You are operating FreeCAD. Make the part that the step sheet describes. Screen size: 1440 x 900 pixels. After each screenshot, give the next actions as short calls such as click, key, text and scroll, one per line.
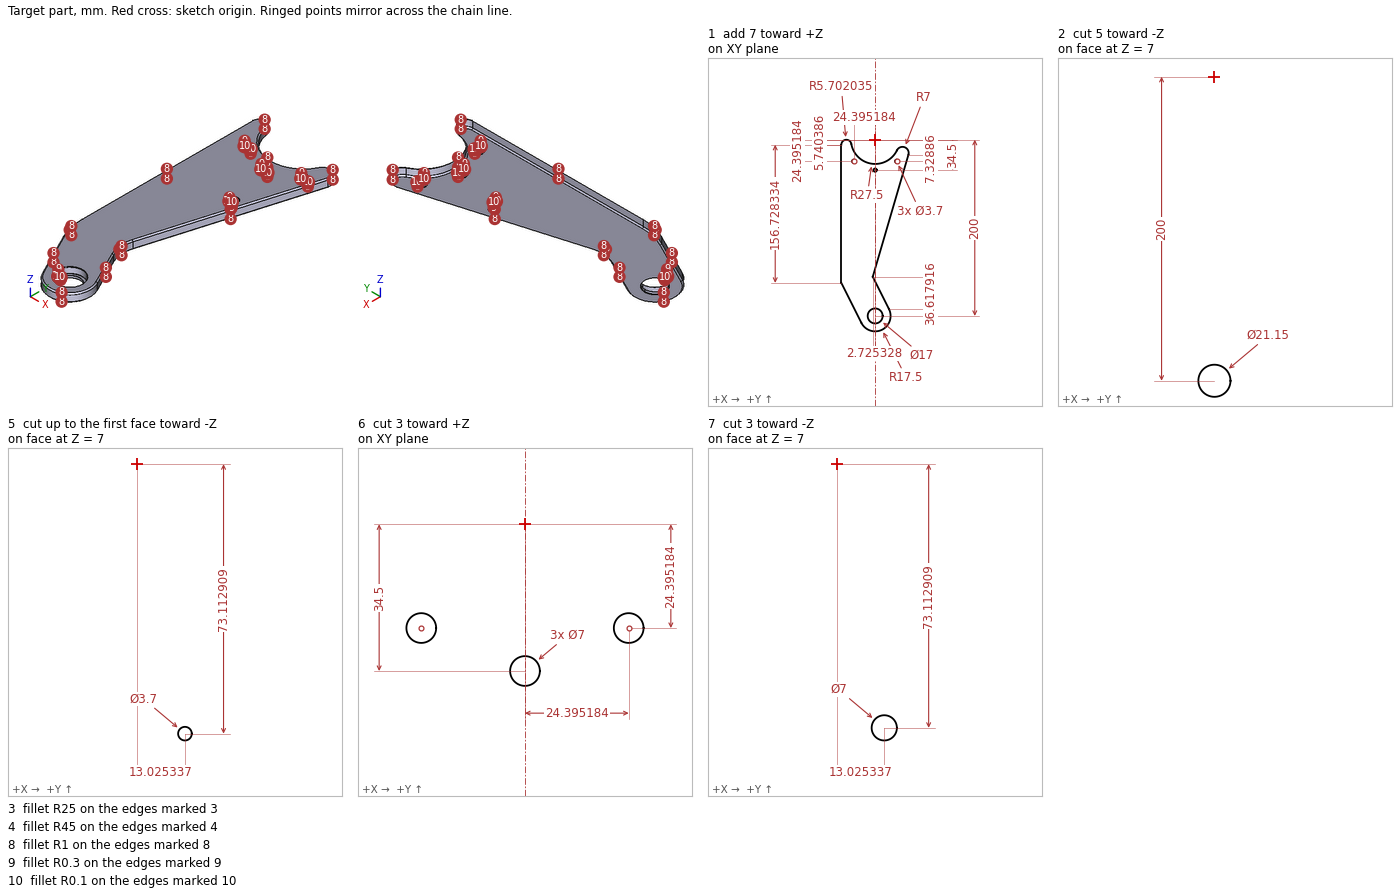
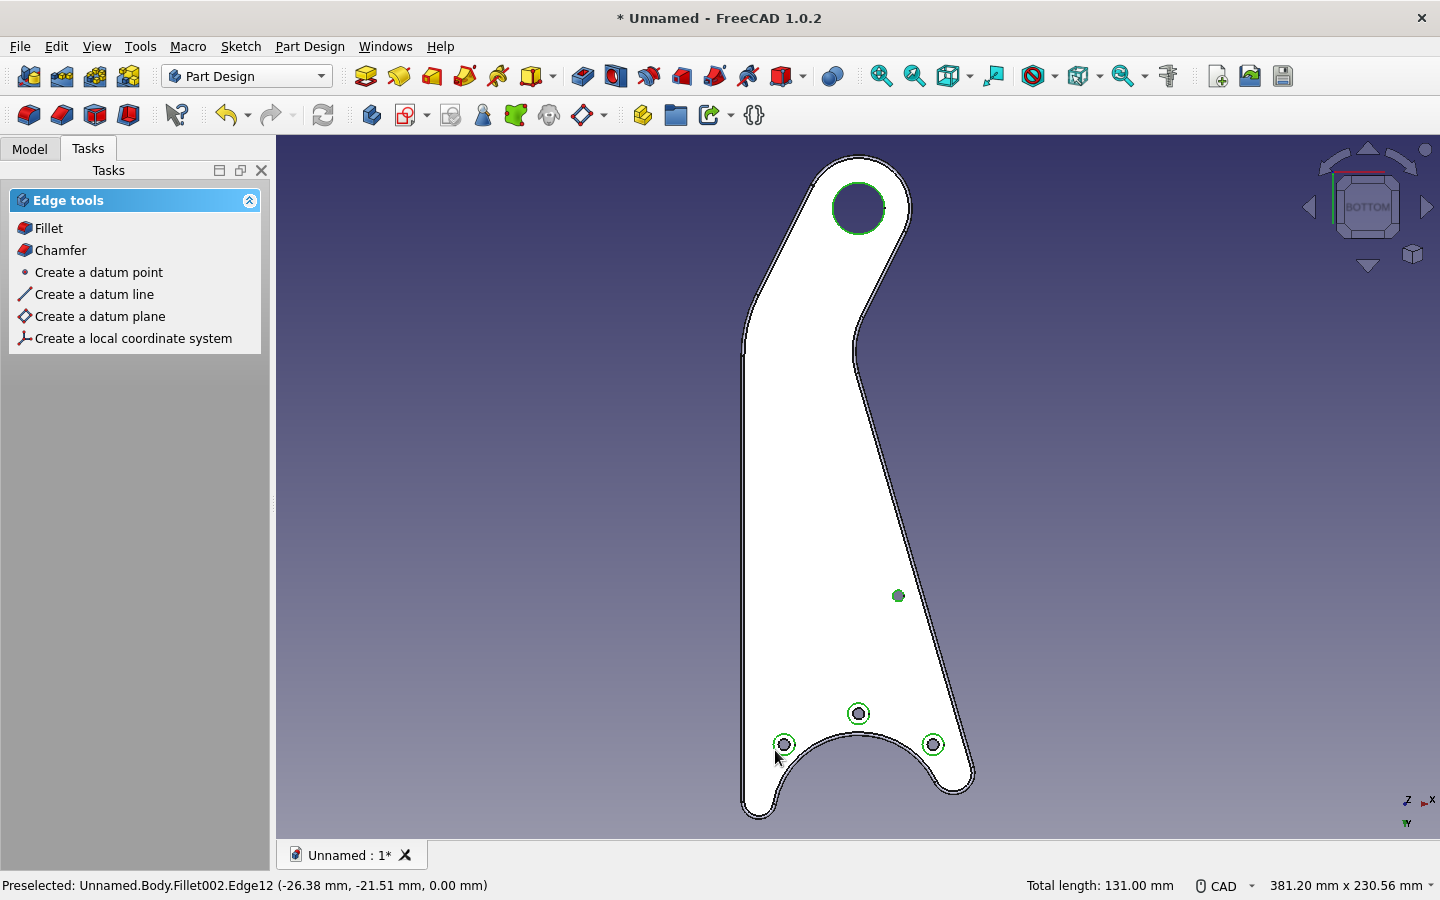
key(0)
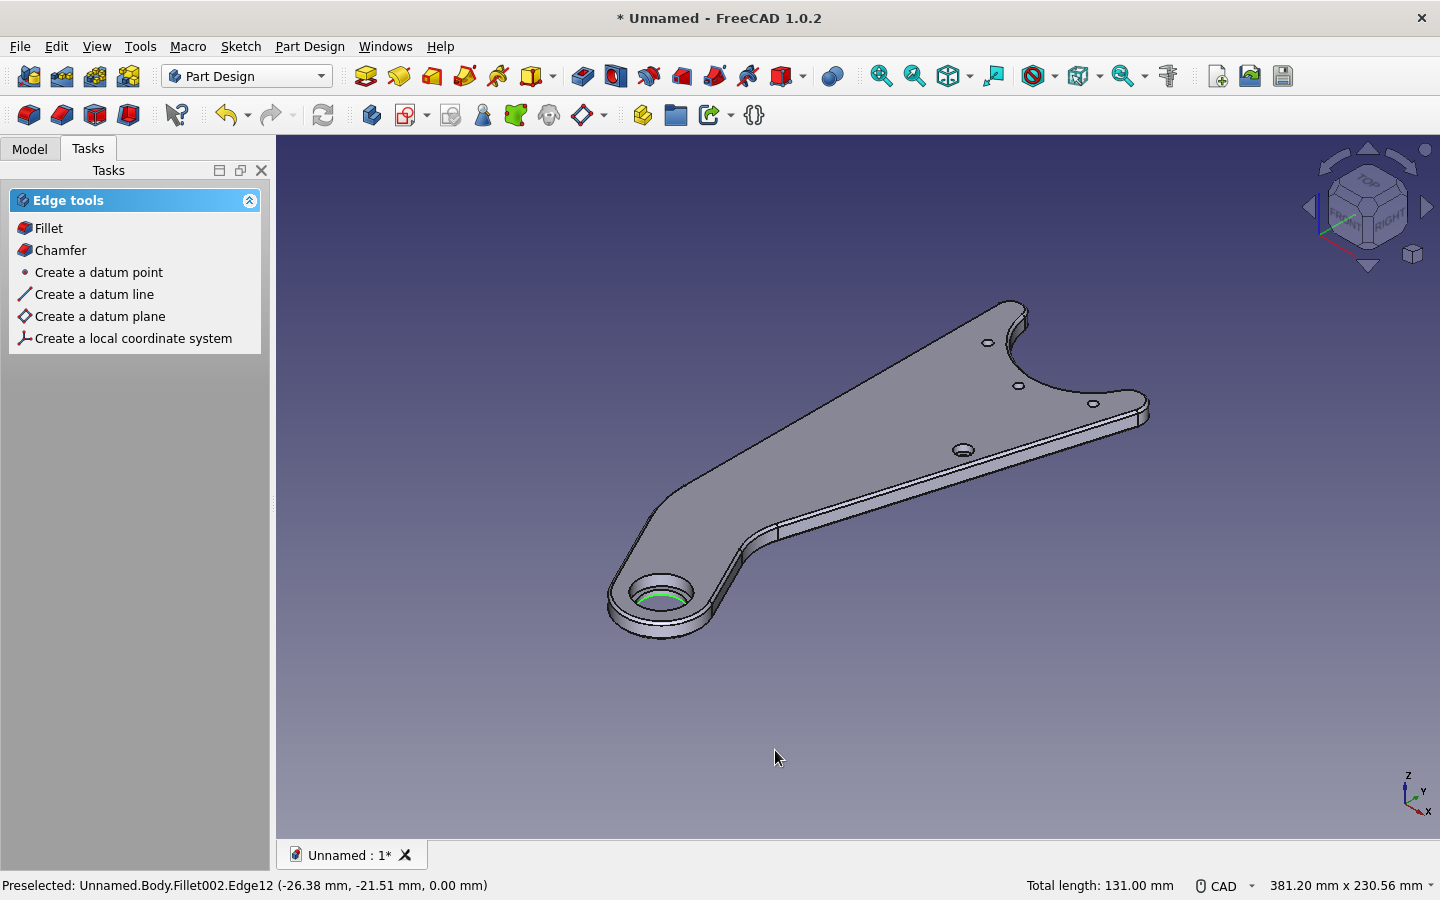
click(984, 340, ctrl)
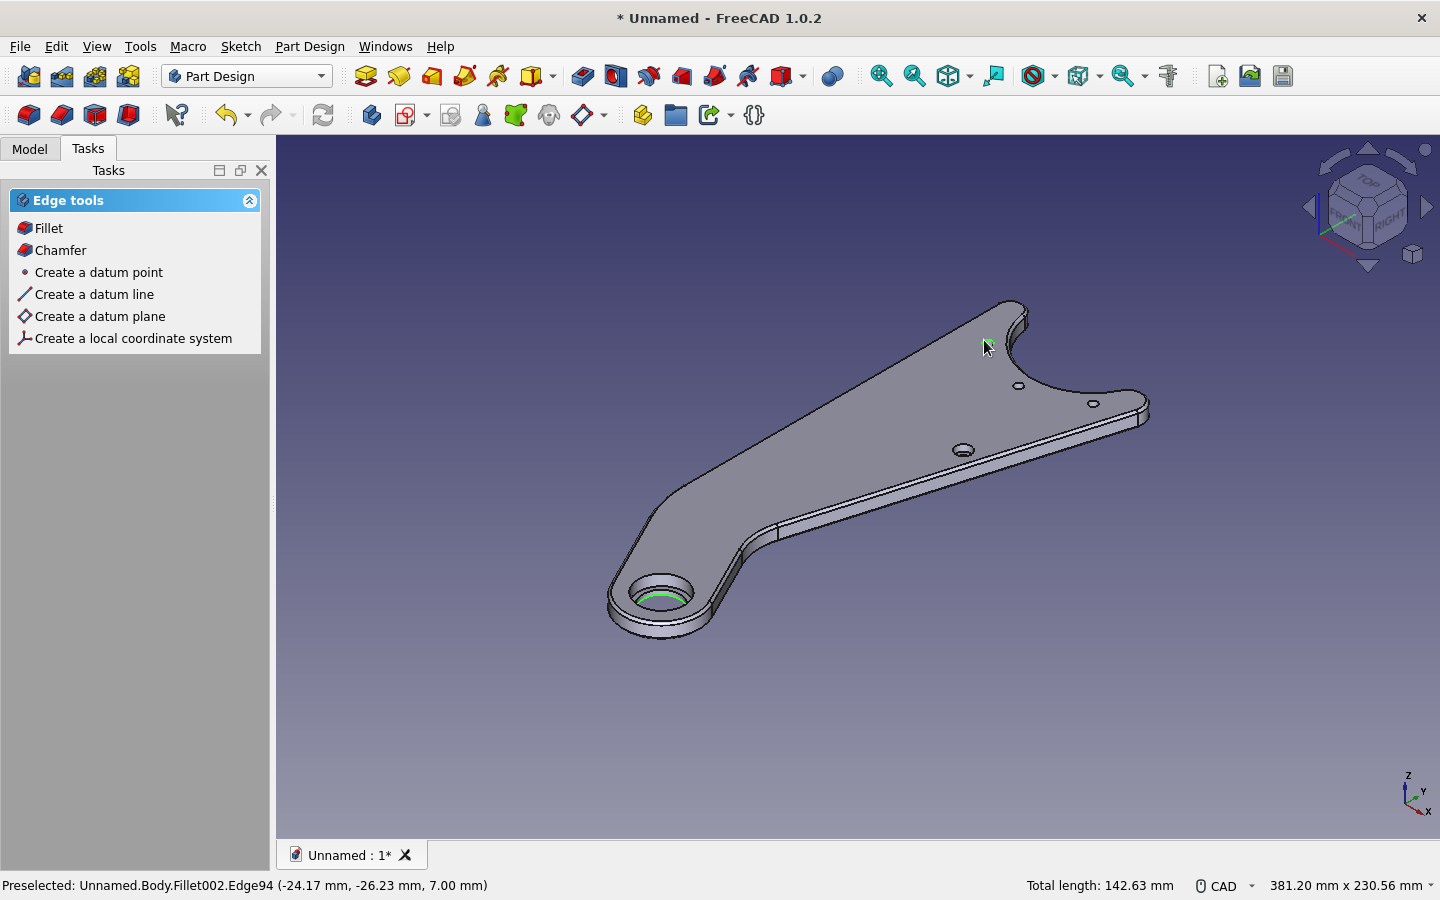
click(1089, 400, ctrl)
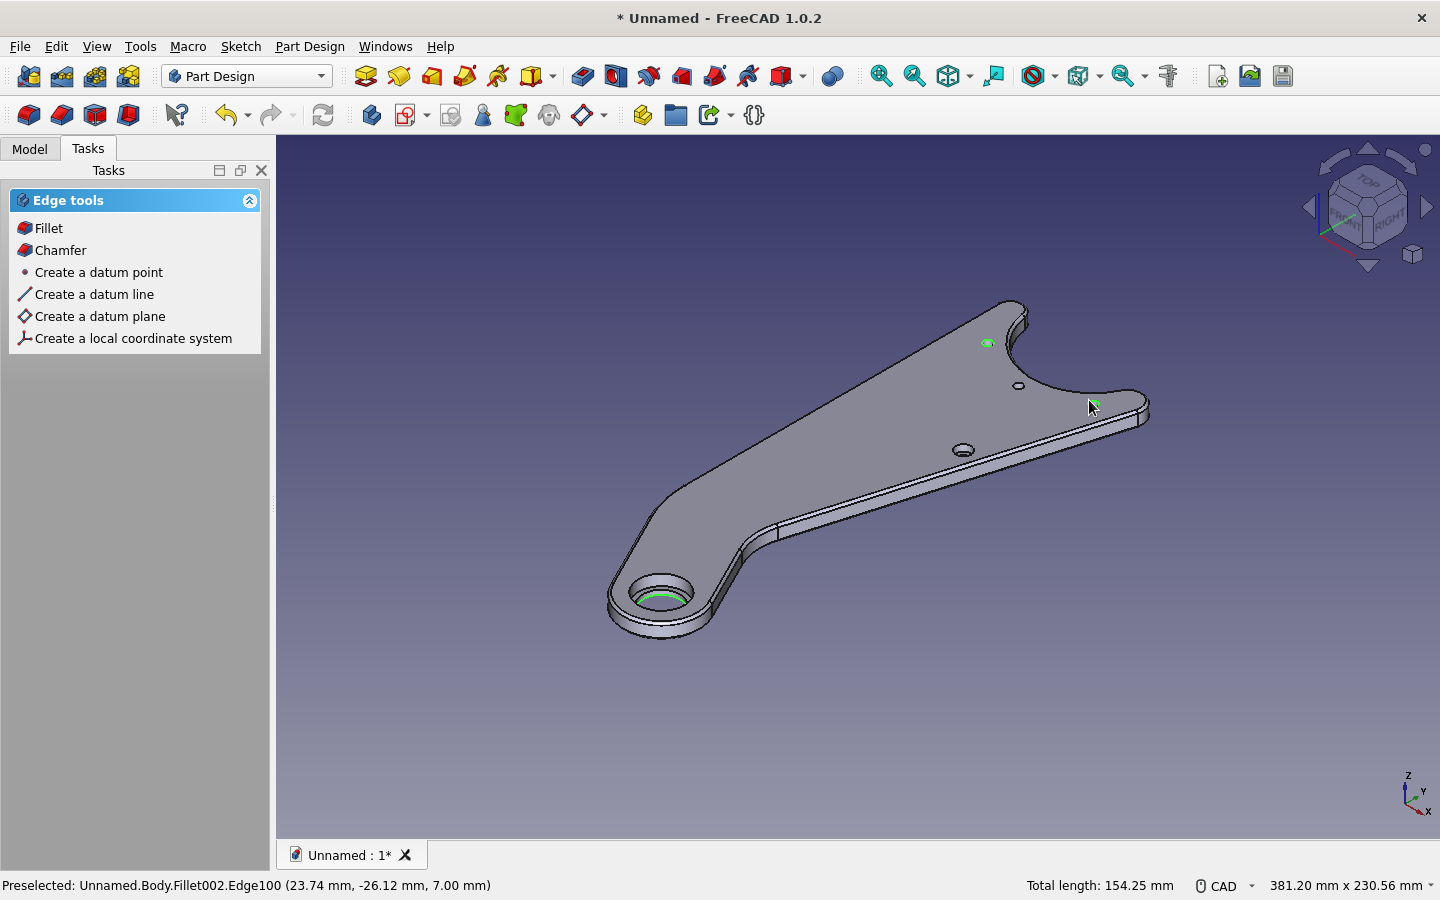
click(1015, 383, ctrl)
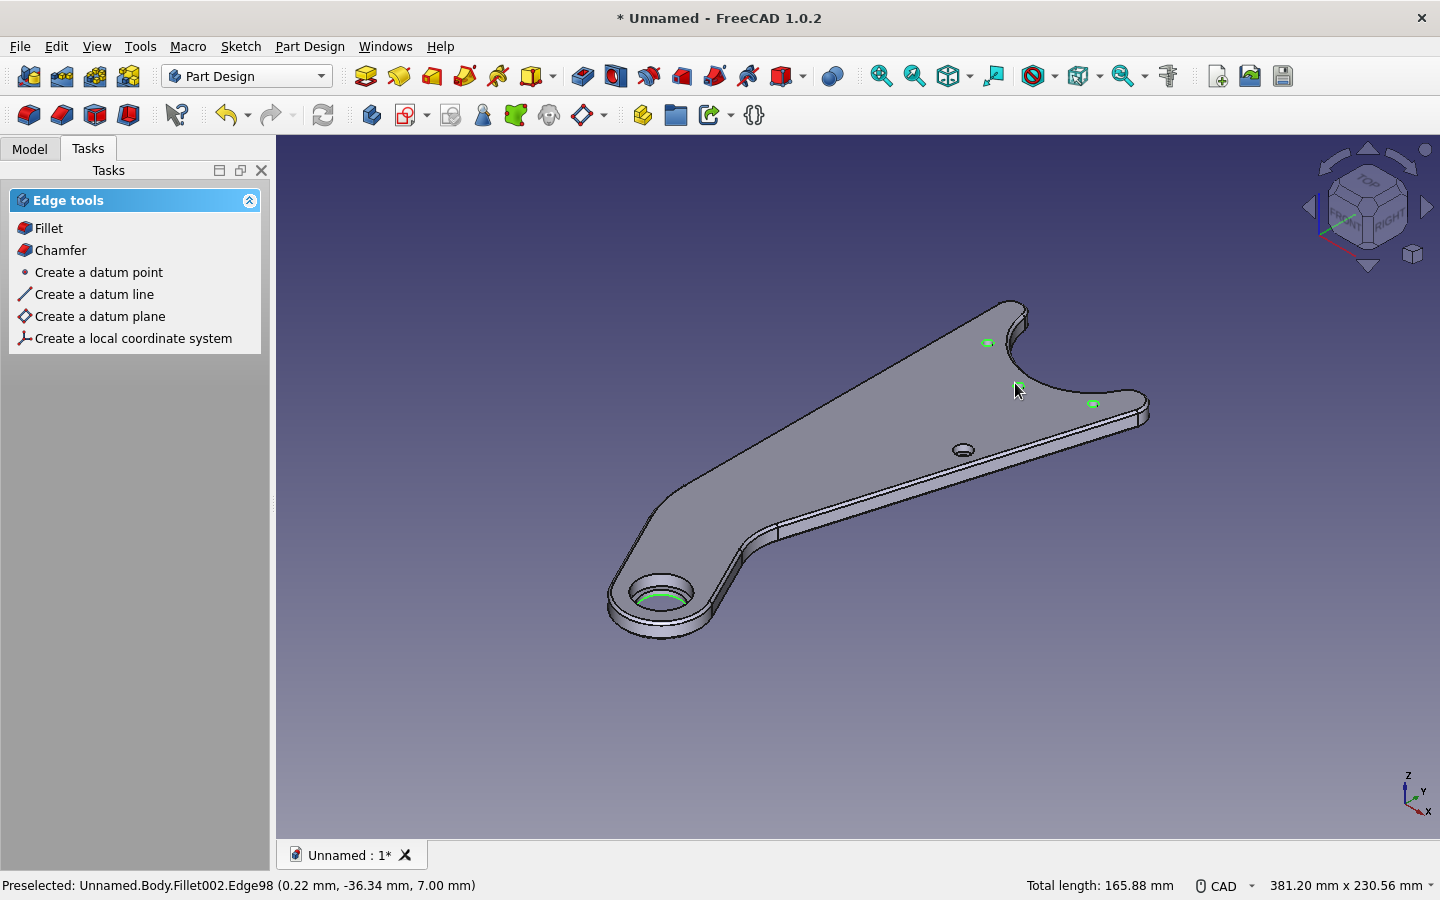
click(639, 578, ctrl)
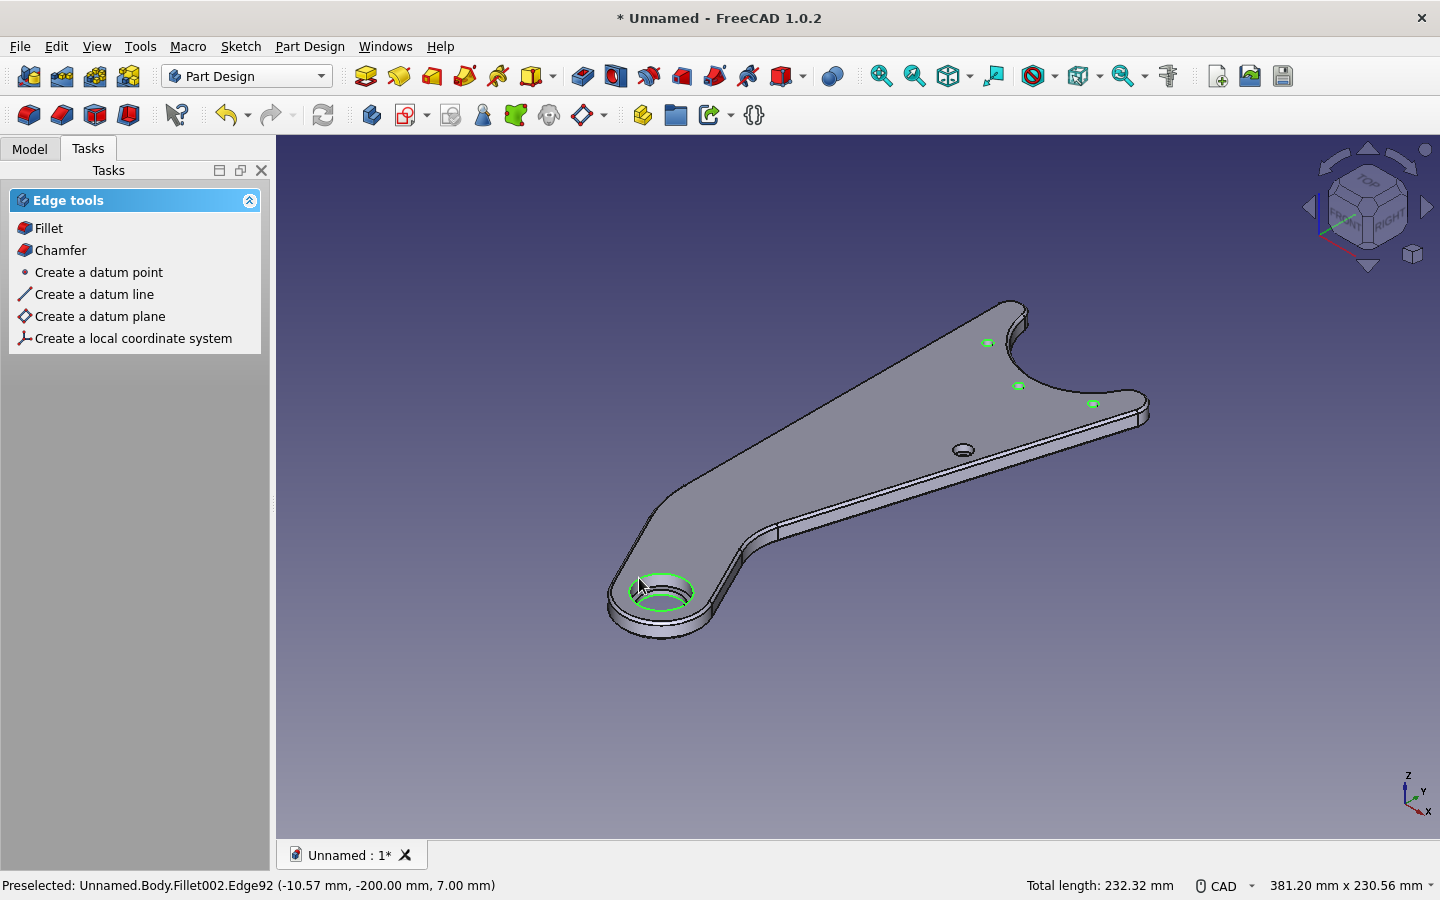
click(956, 445, ctrl)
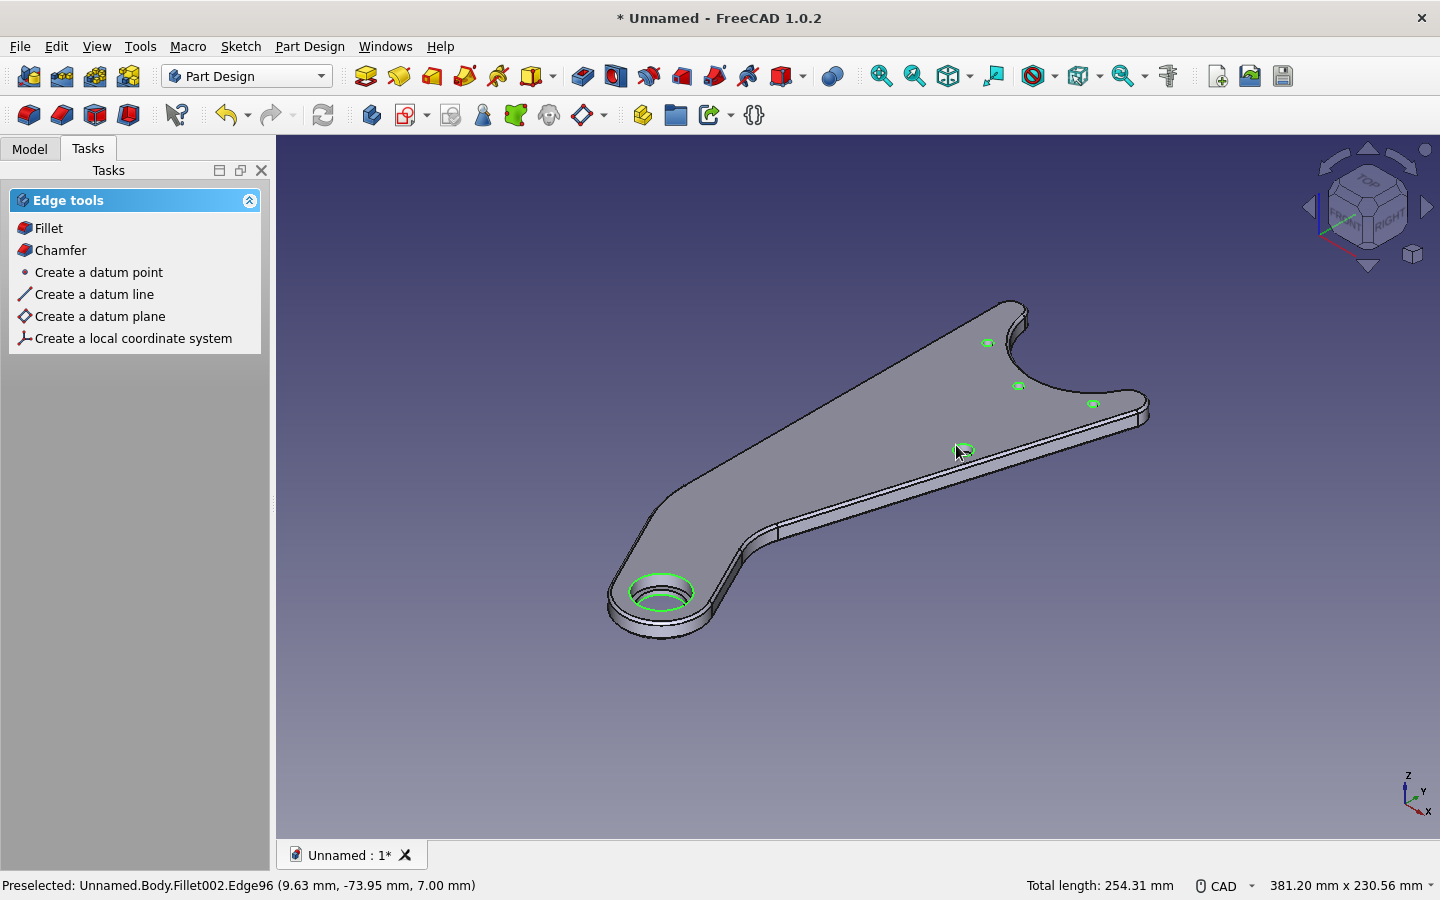
click(29, 116)